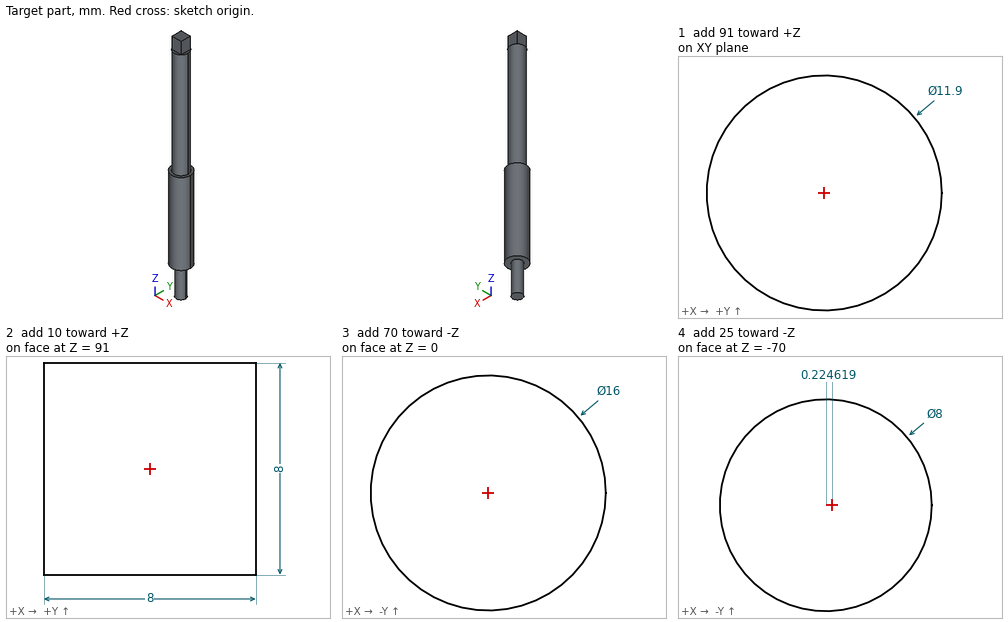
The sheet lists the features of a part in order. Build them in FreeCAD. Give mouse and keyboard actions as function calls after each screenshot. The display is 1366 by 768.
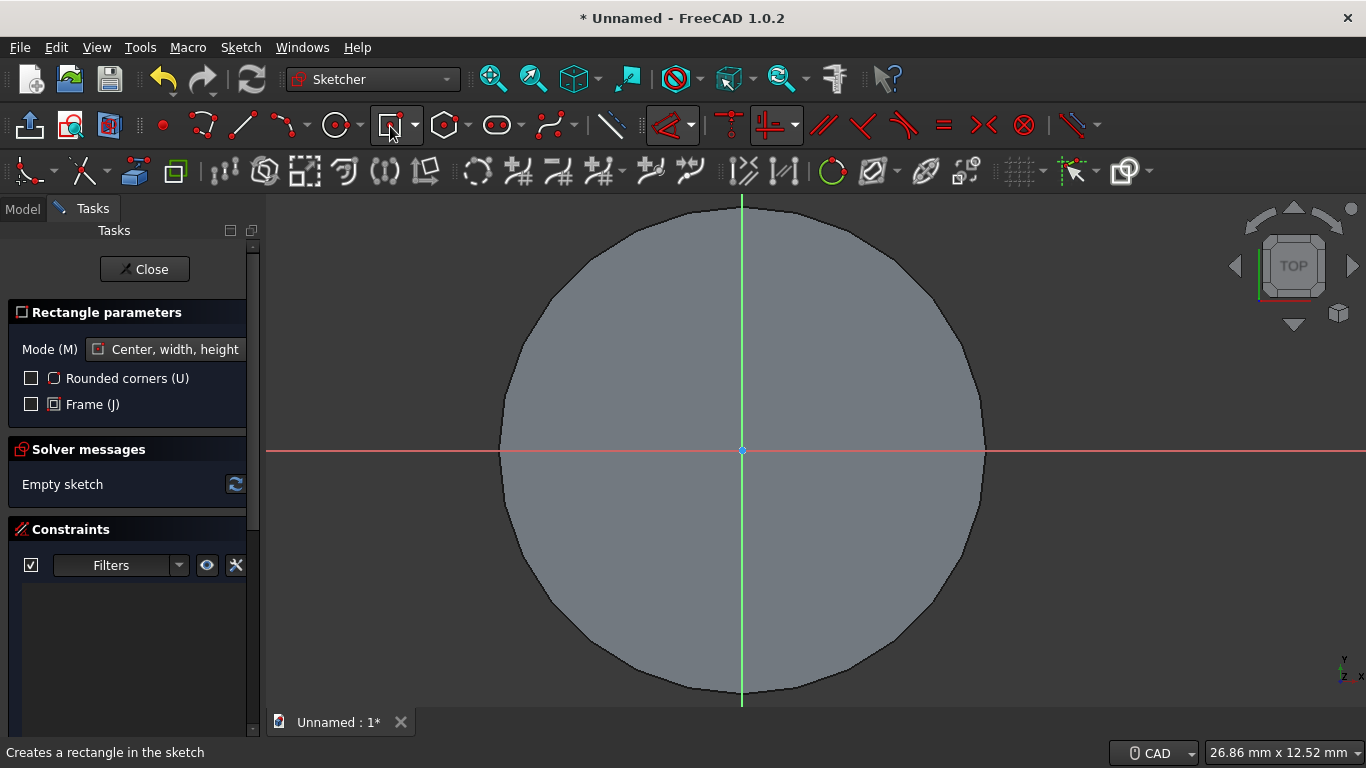
click(742, 450)
click(906, 287)
key(Escape)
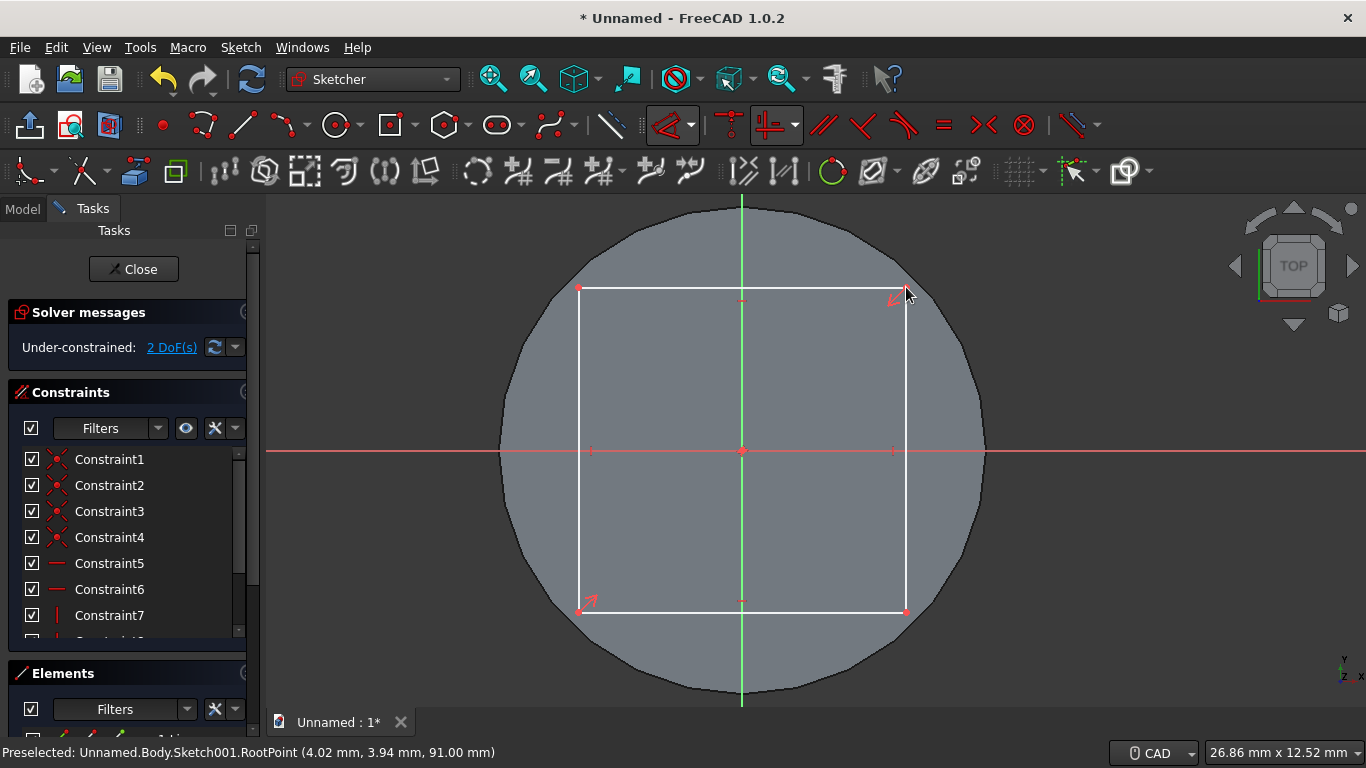
click(677, 613)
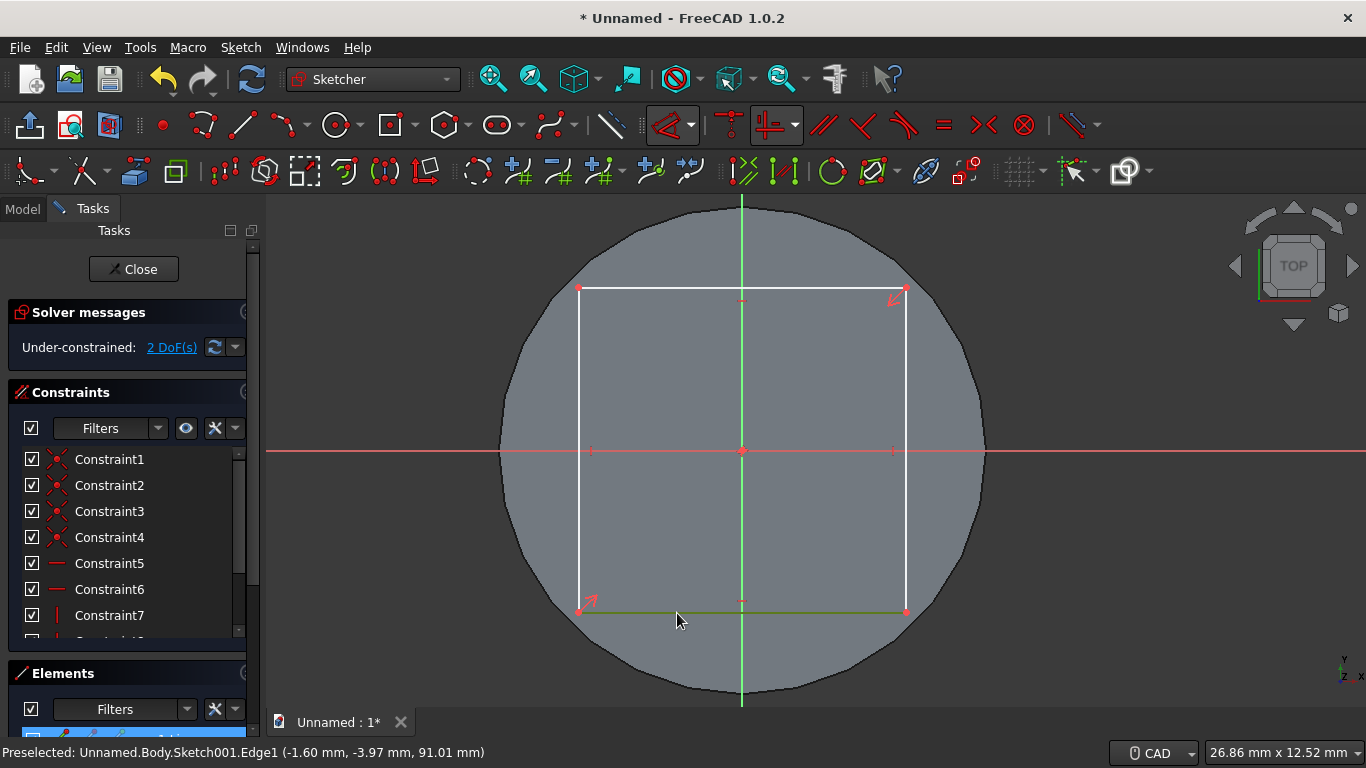
key(l)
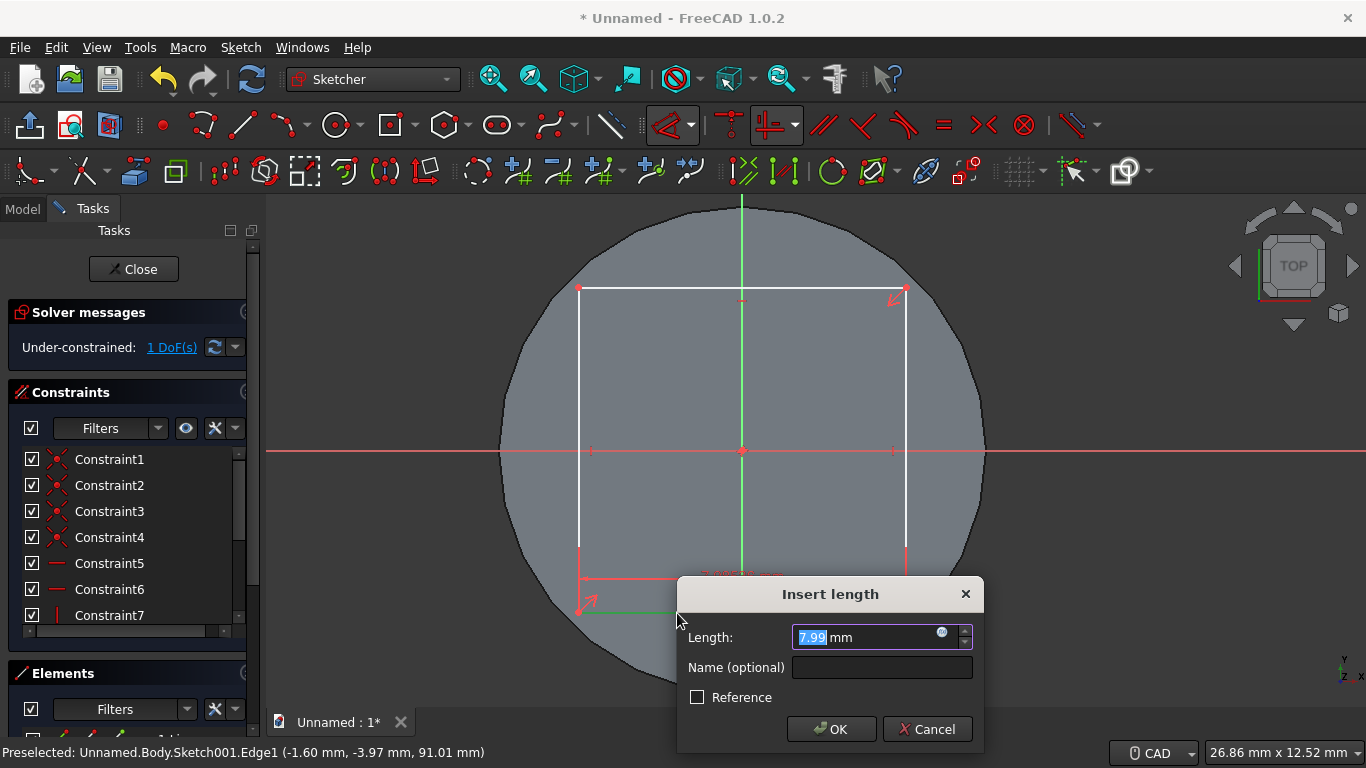
text(8)
key(Return)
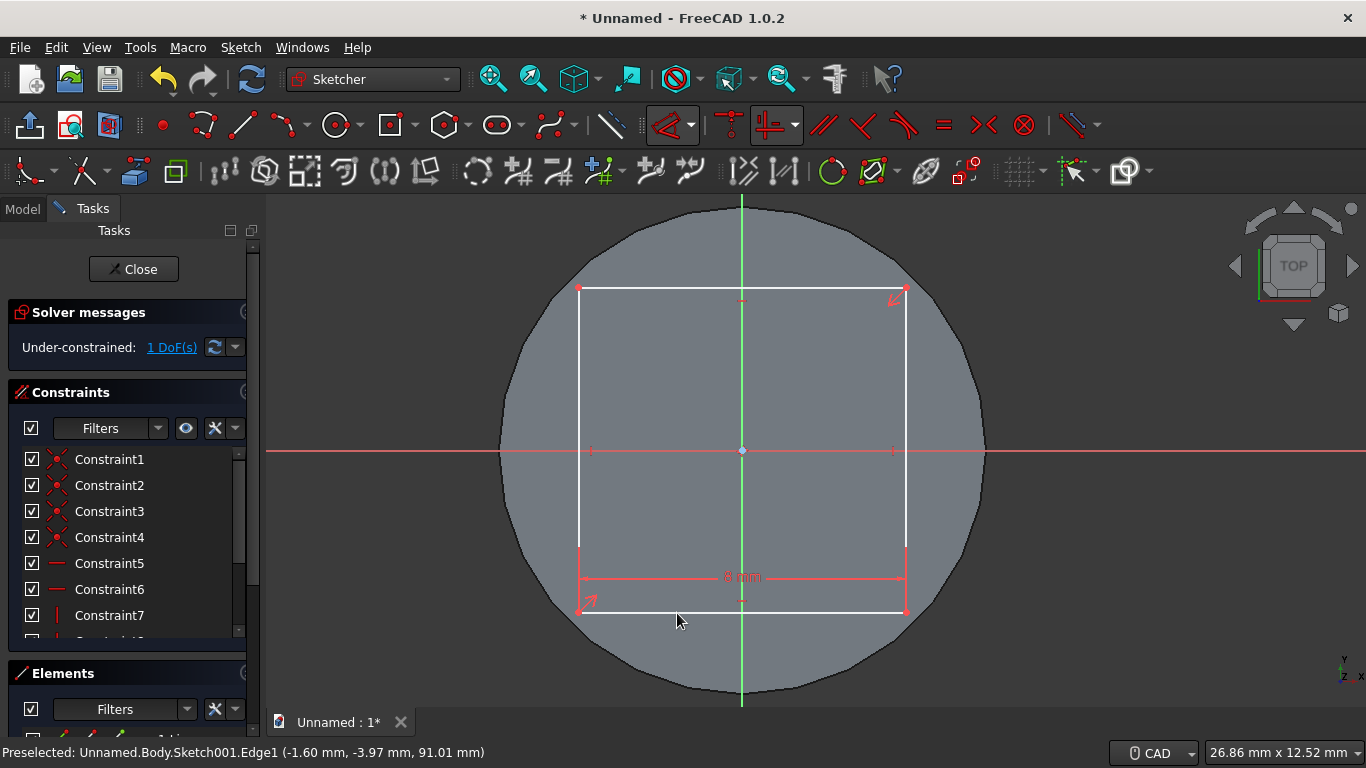
click(906, 516)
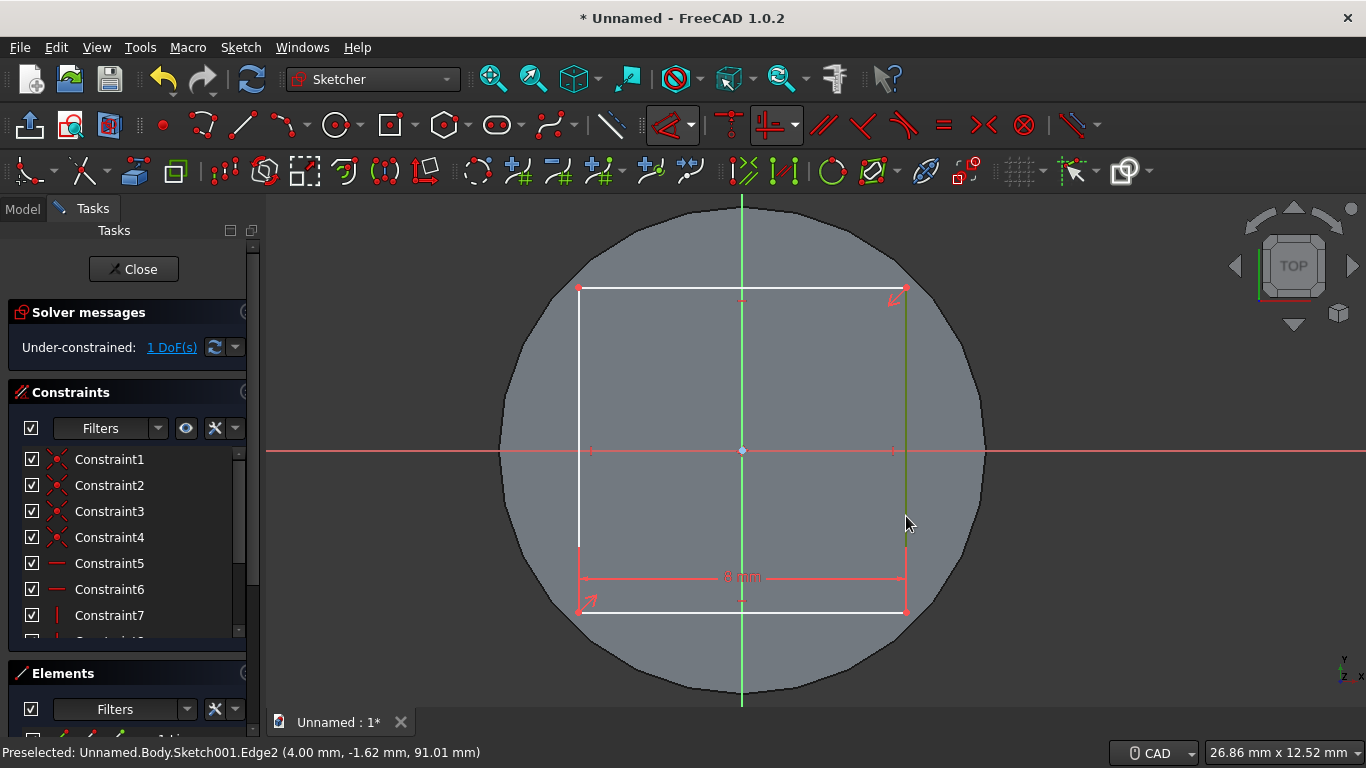
click(694, 126)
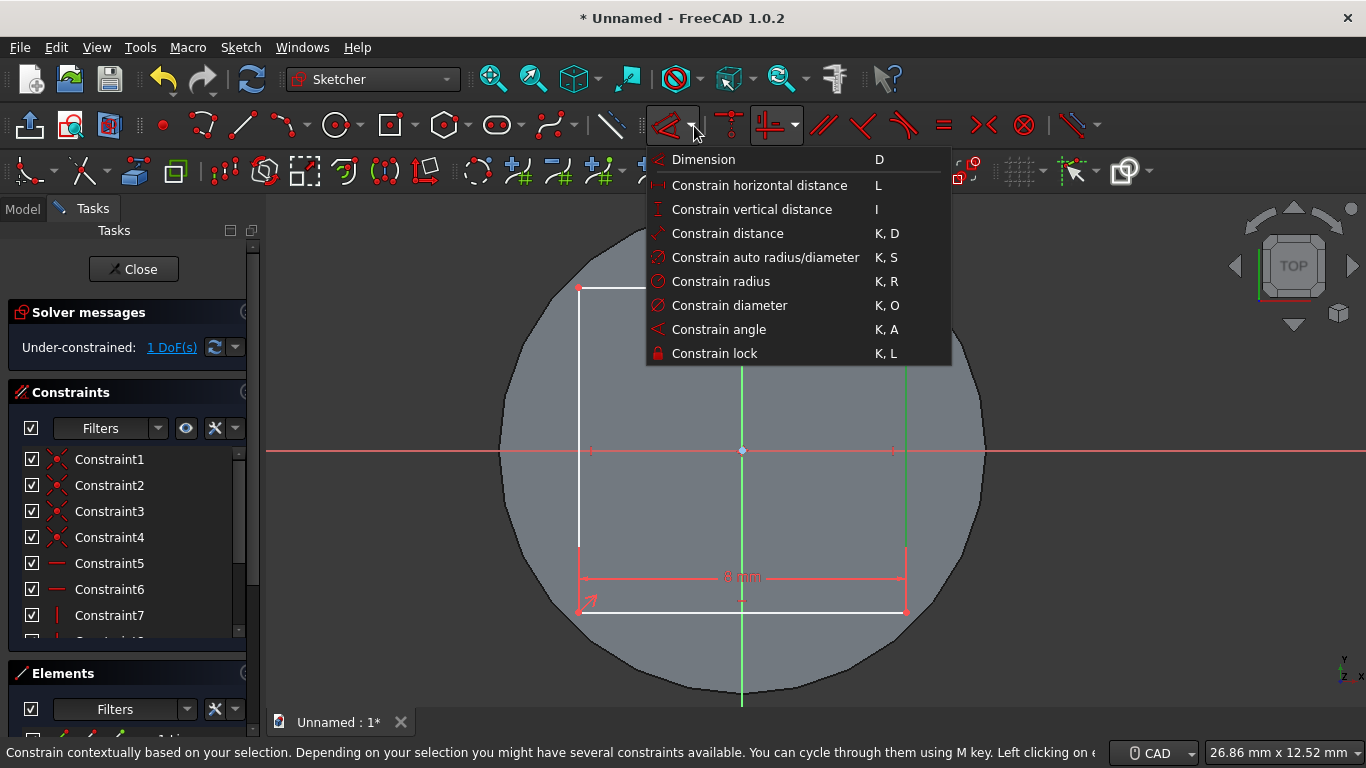
click(799, 209)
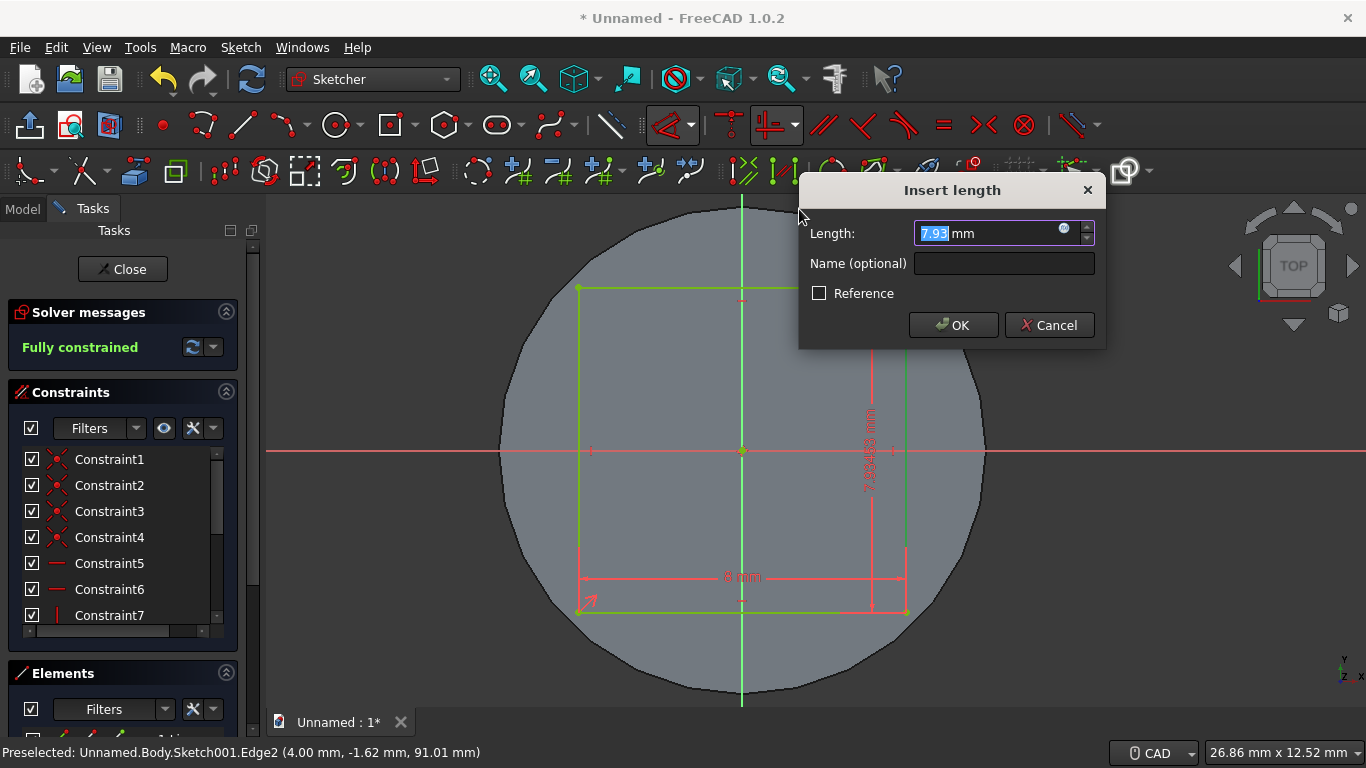
text(8)
key(Return)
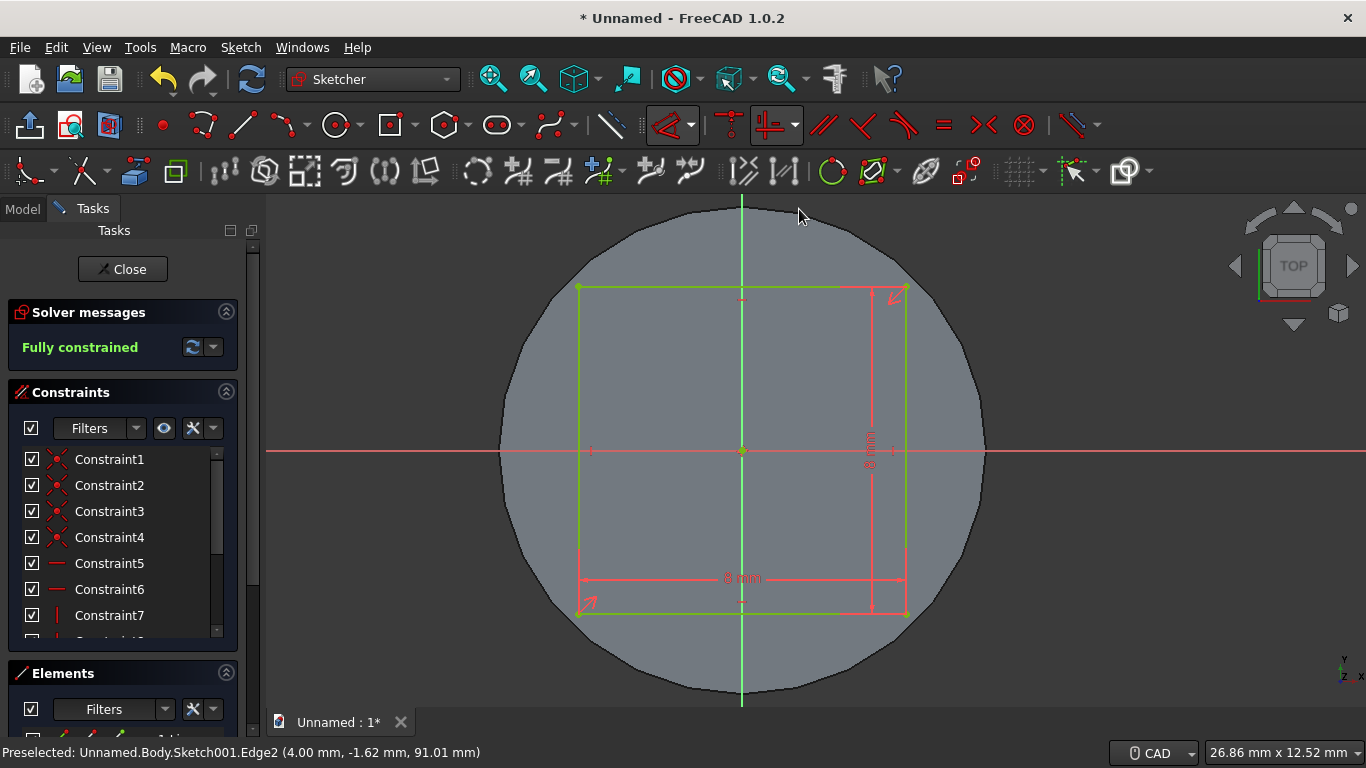
click(123, 269)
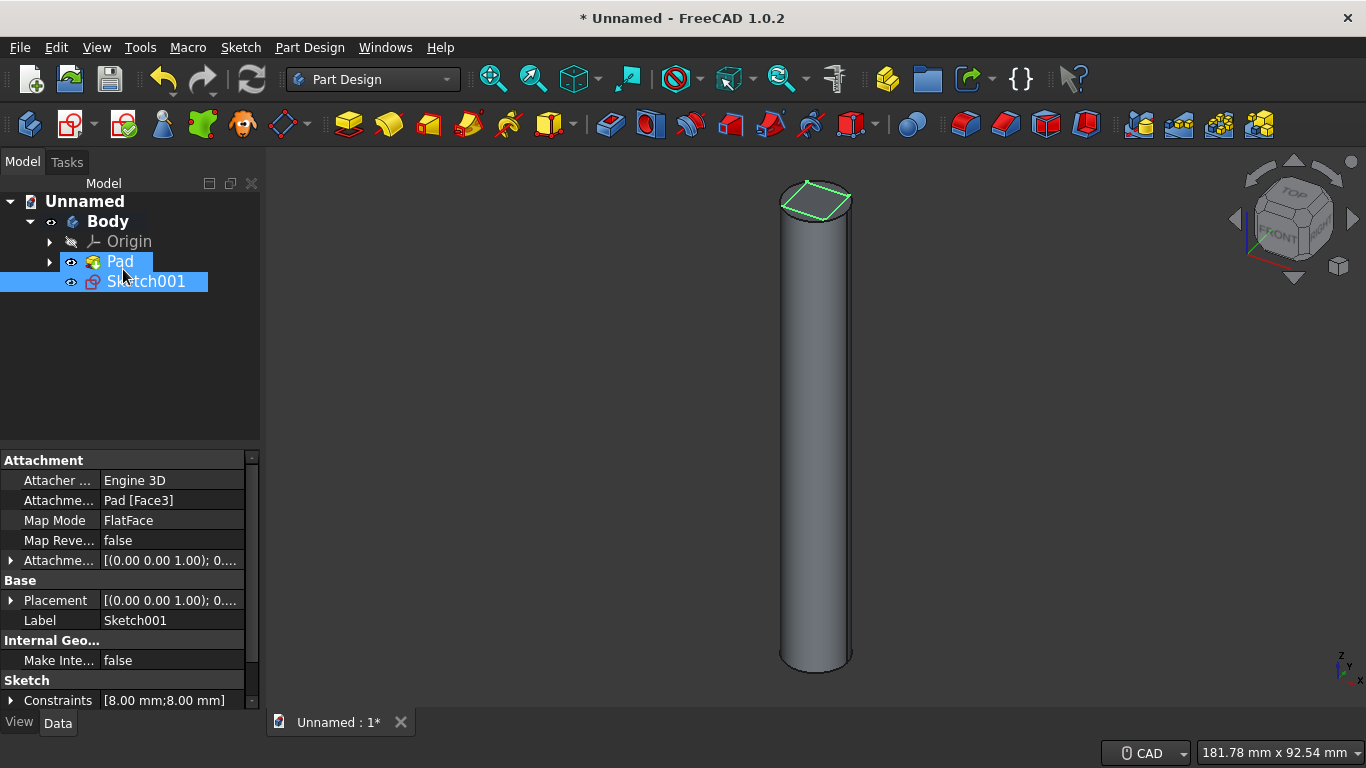
click(350, 124)